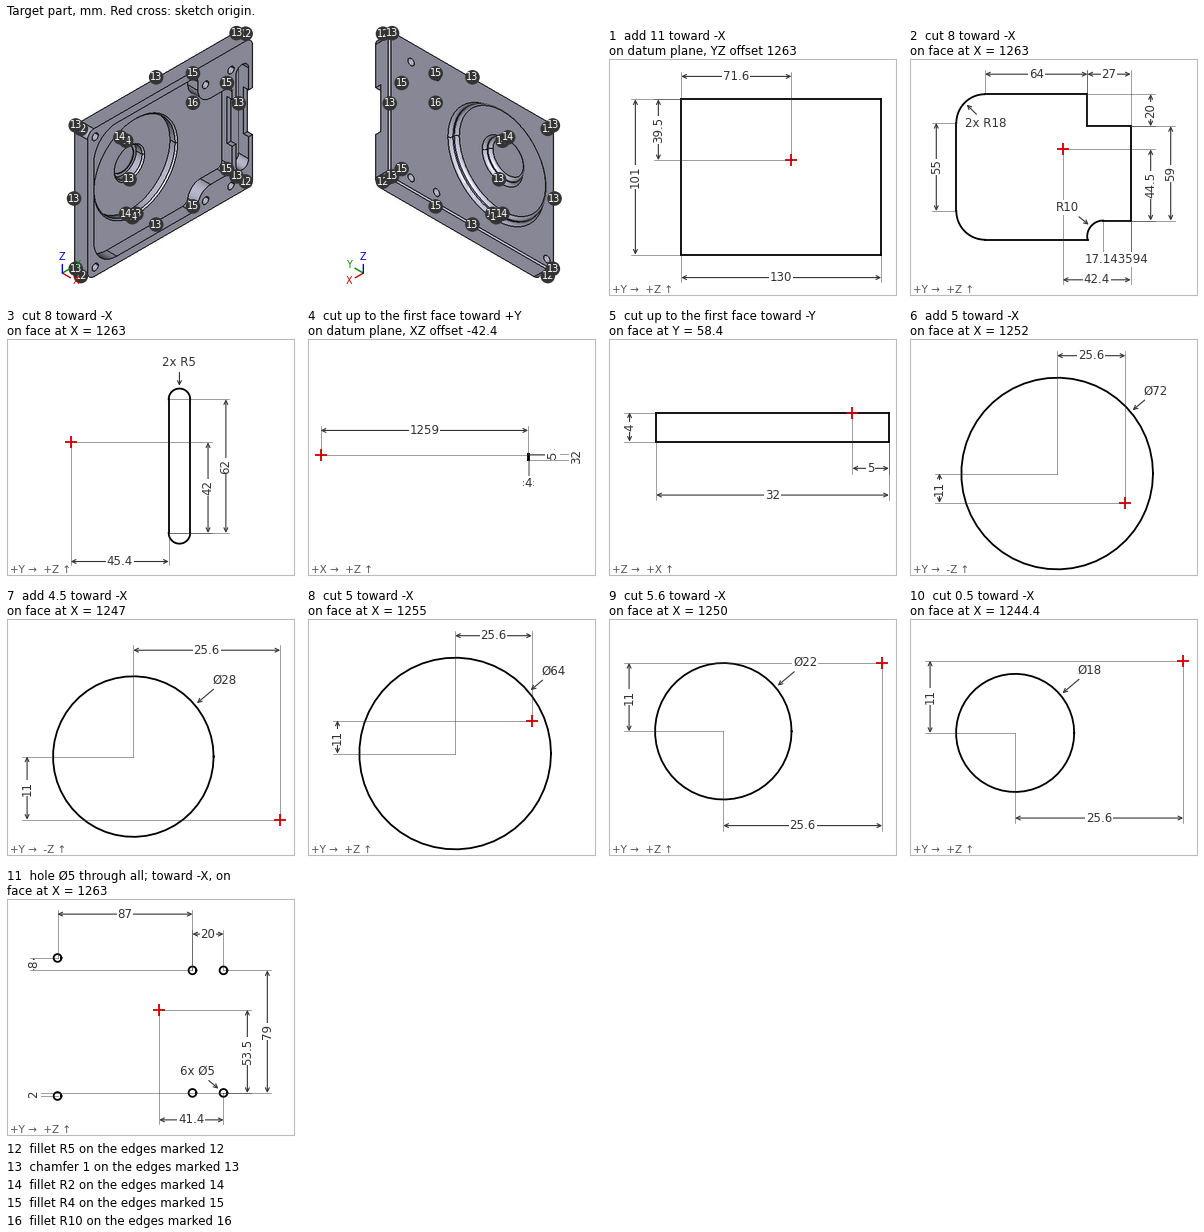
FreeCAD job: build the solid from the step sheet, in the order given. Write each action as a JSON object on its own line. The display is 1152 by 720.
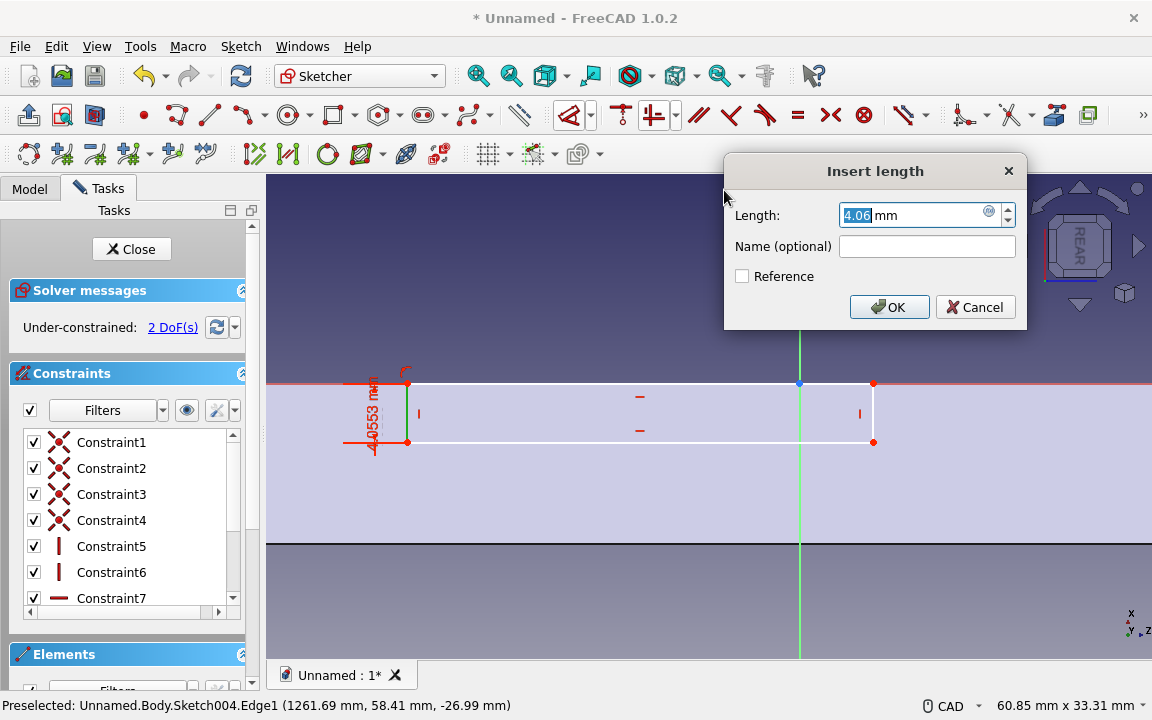
{"action": "type", "text": "4"}
{"action": "key", "text": "Return"}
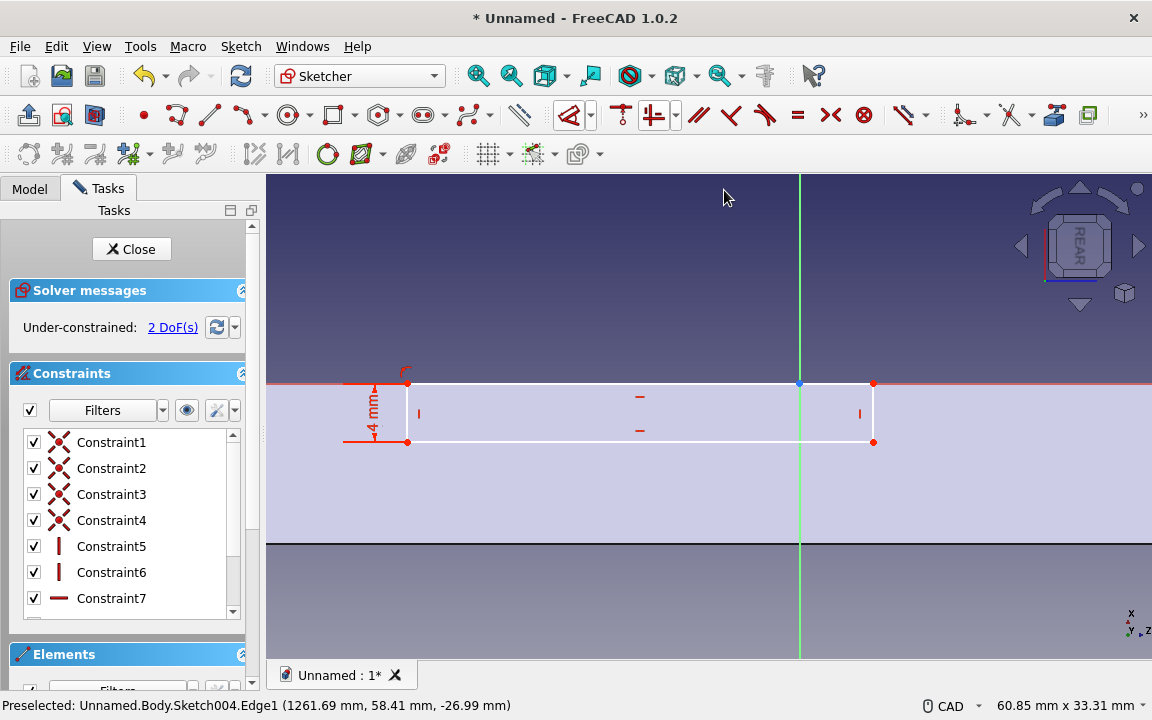
{"action": "left_click", "coordinate": [547, 442]}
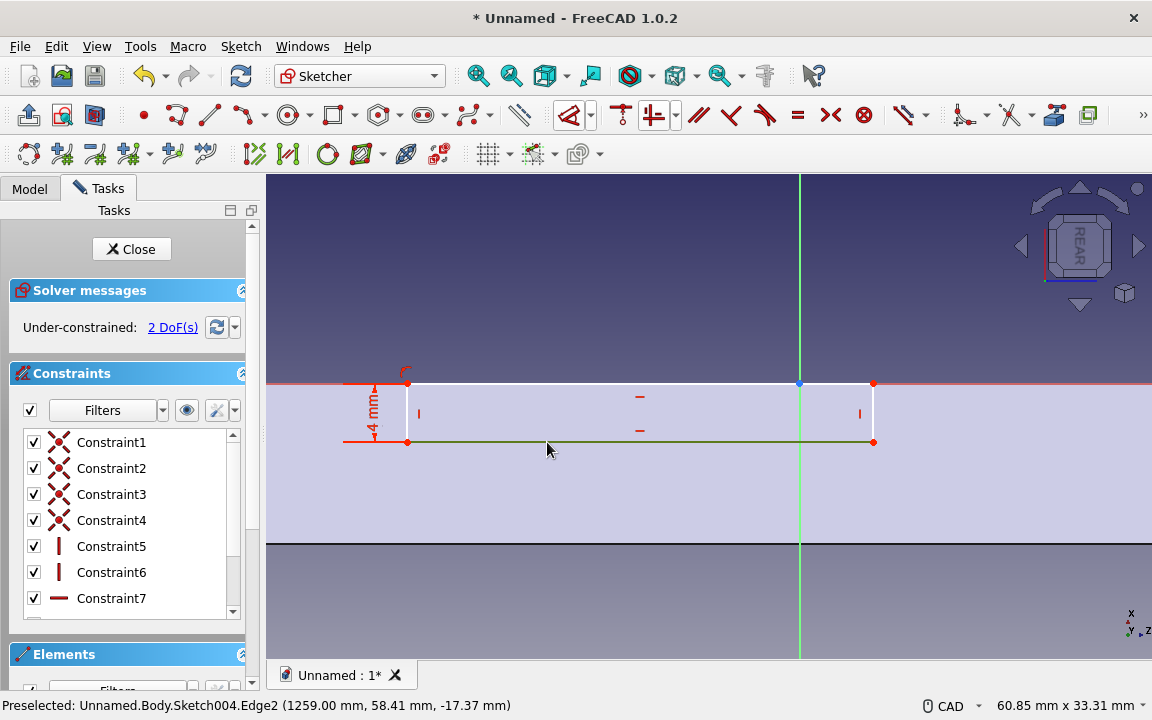
{"action": "key", "text": "l"}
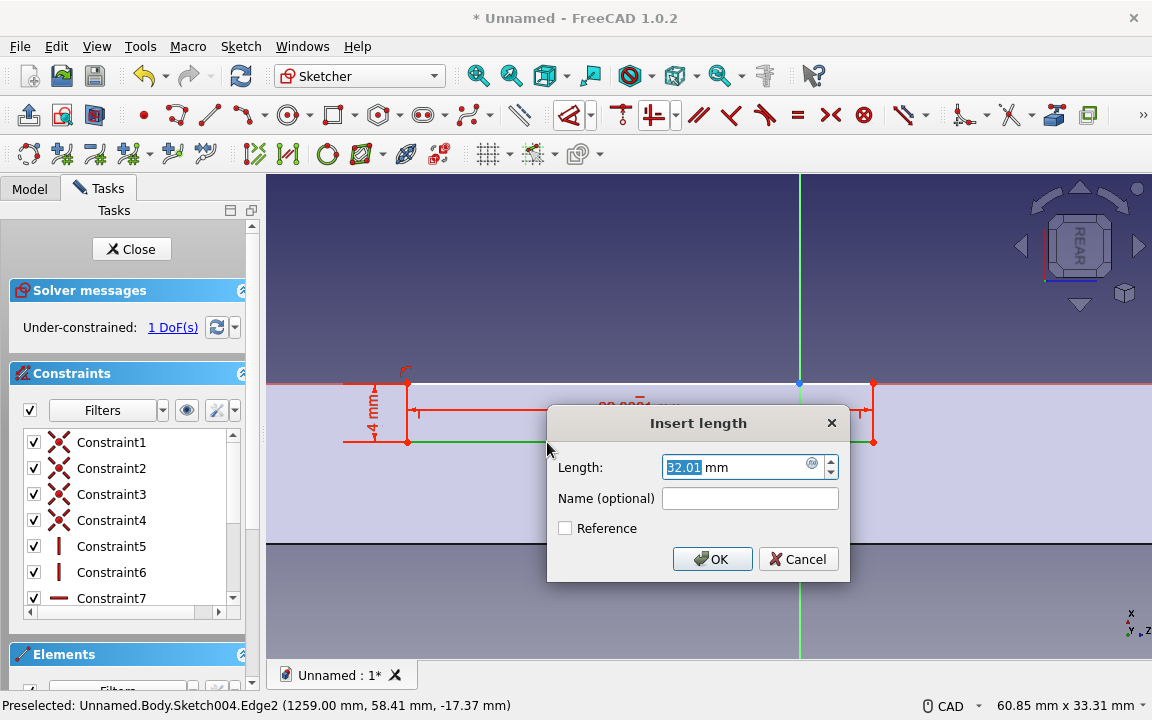
{"action": "type", "text": "32"}
{"action": "key", "text": "Return"}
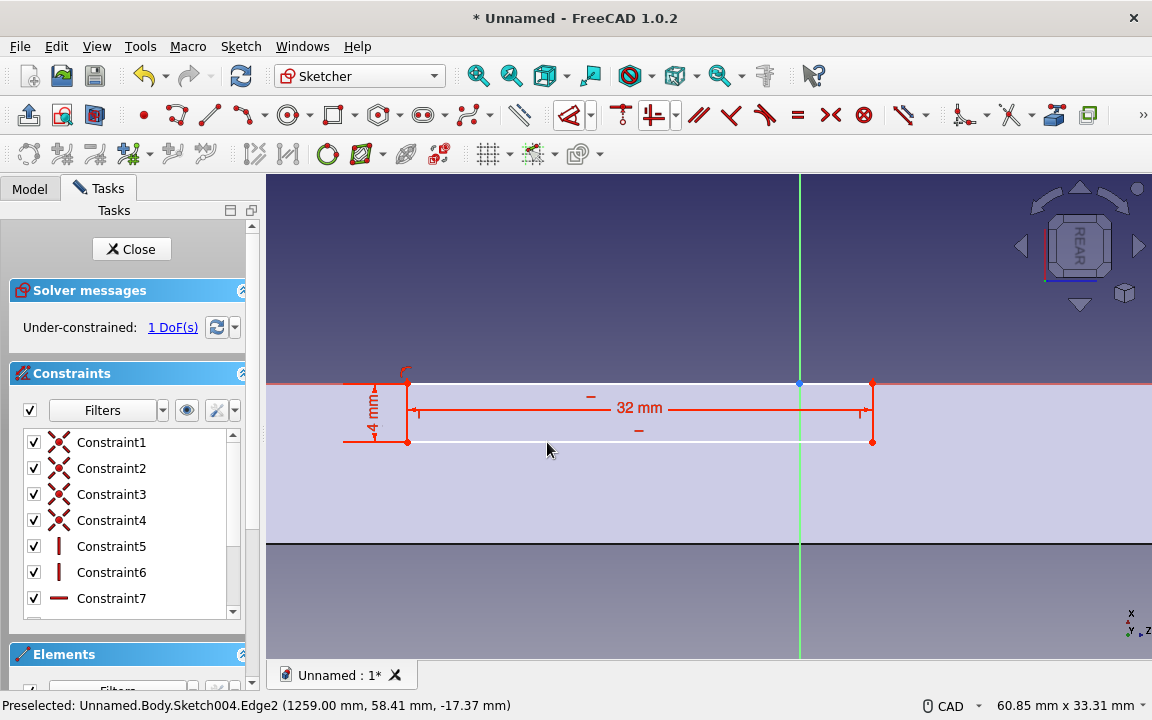
{"action": "left_click", "coordinate": [873, 442]}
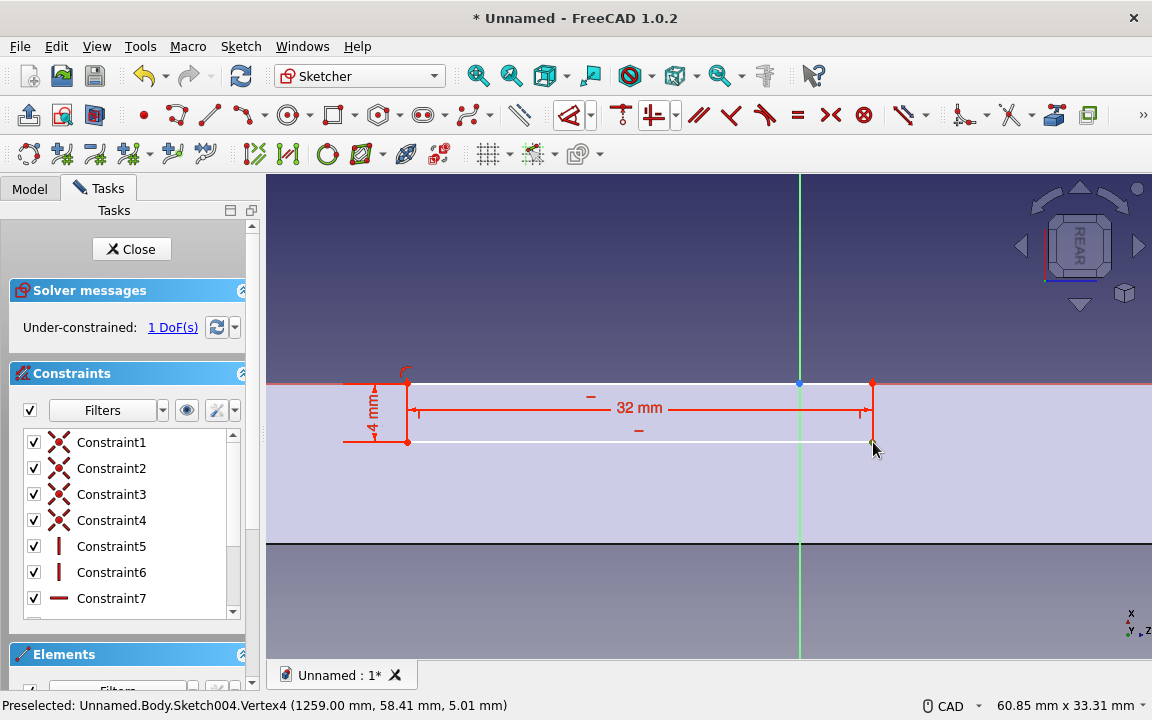
{"action": "key", "text": "l"}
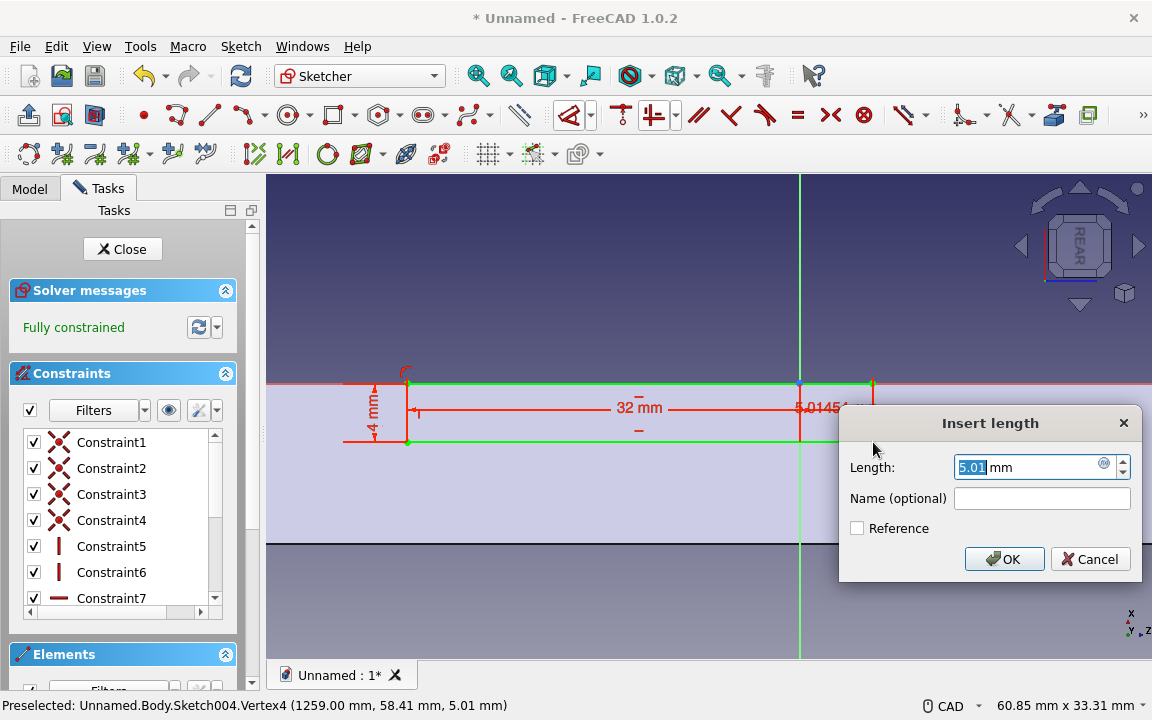
{"action": "type", "text": "5"}
{"action": "key", "text": "Return"}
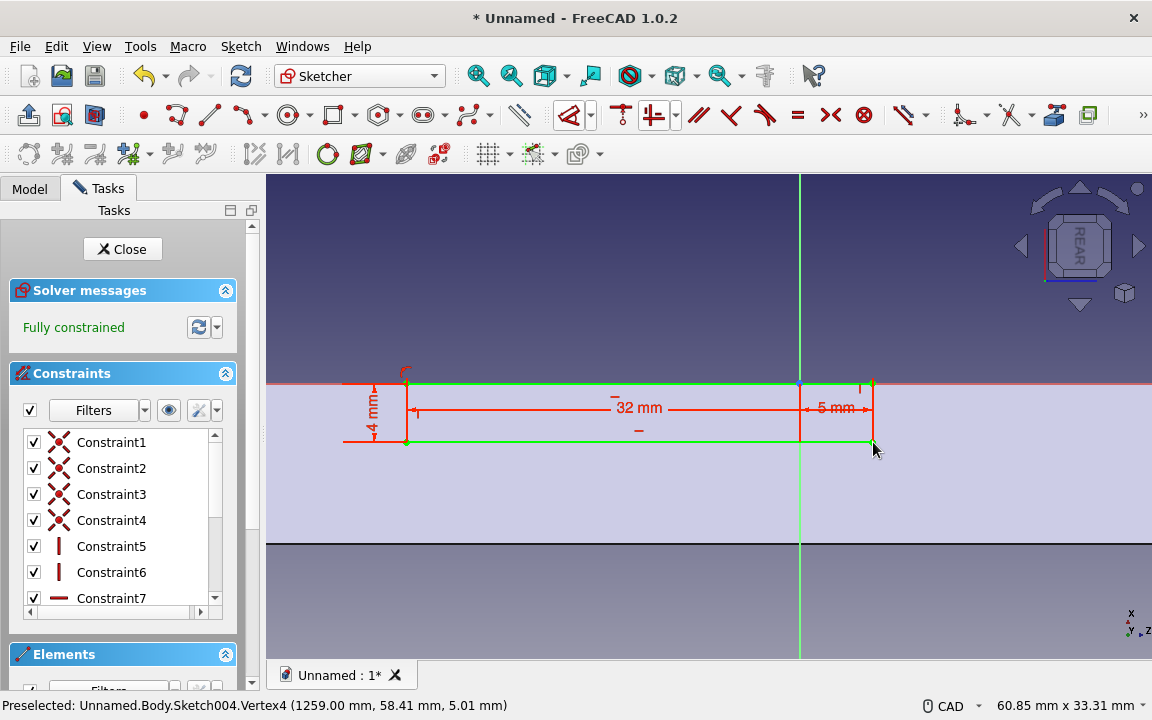
{"action": "left_click", "coordinate": [123, 249]}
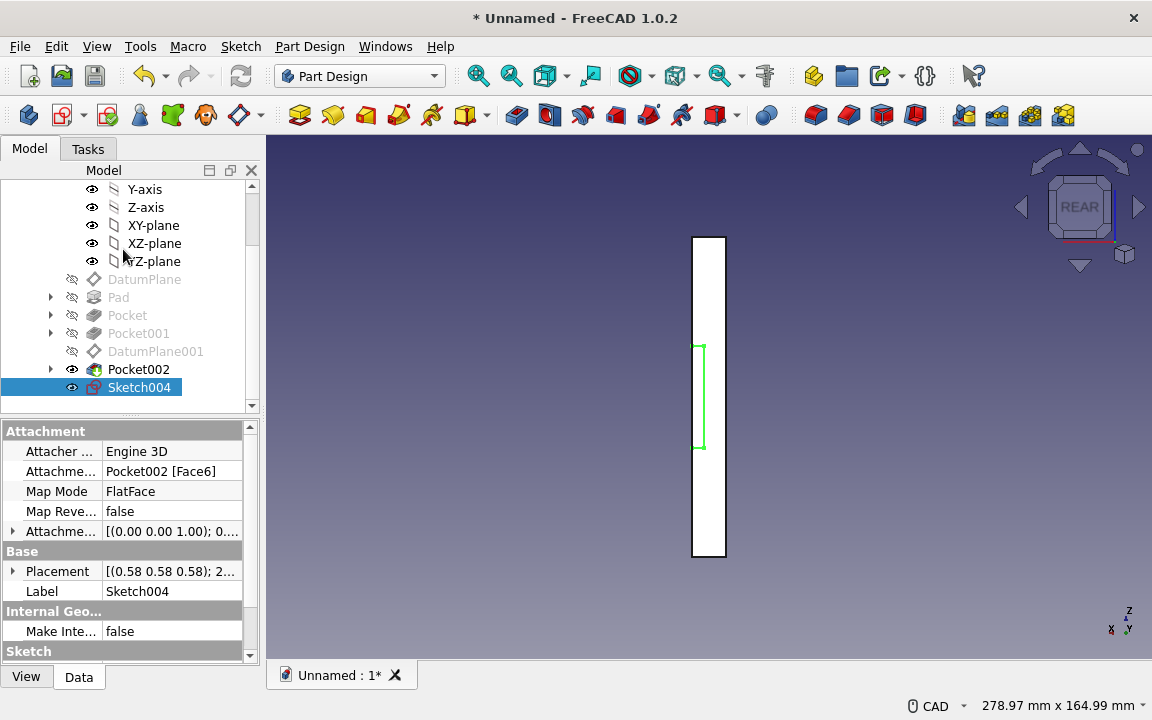
{"action": "left_click", "coordinate": [517, 116]}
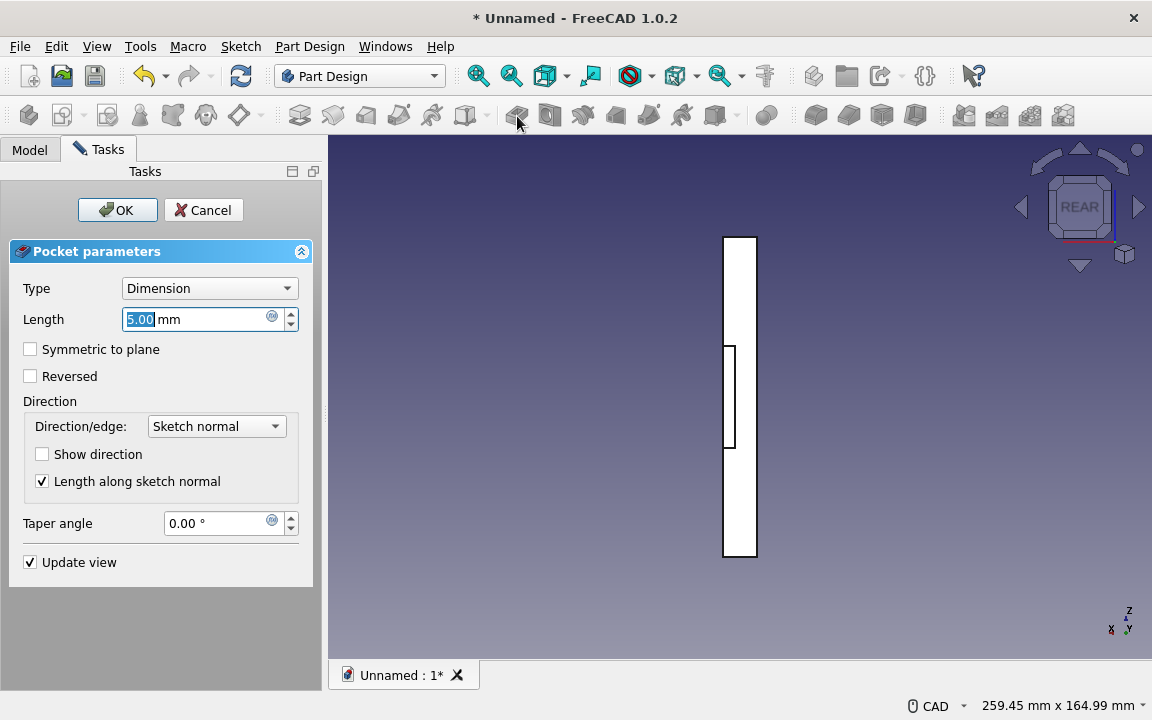
{"action": "left_click", "coordinate": [210, 288]}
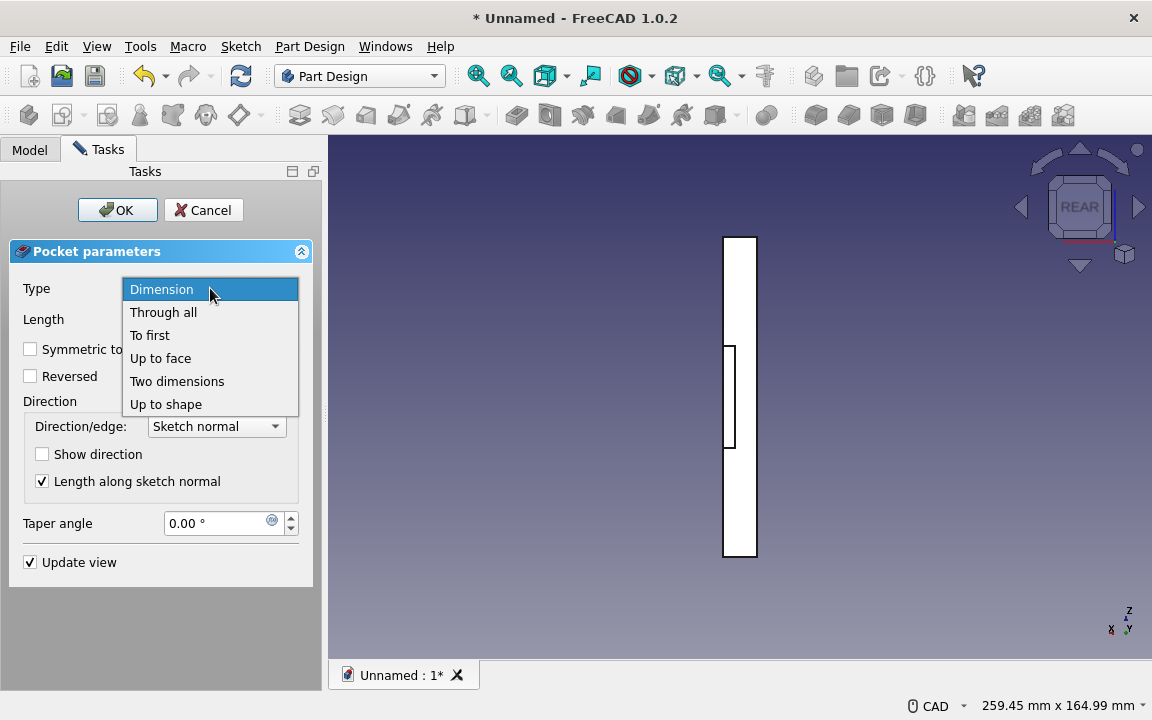
{"action": "left_click", "coordinate": [208, 336]}